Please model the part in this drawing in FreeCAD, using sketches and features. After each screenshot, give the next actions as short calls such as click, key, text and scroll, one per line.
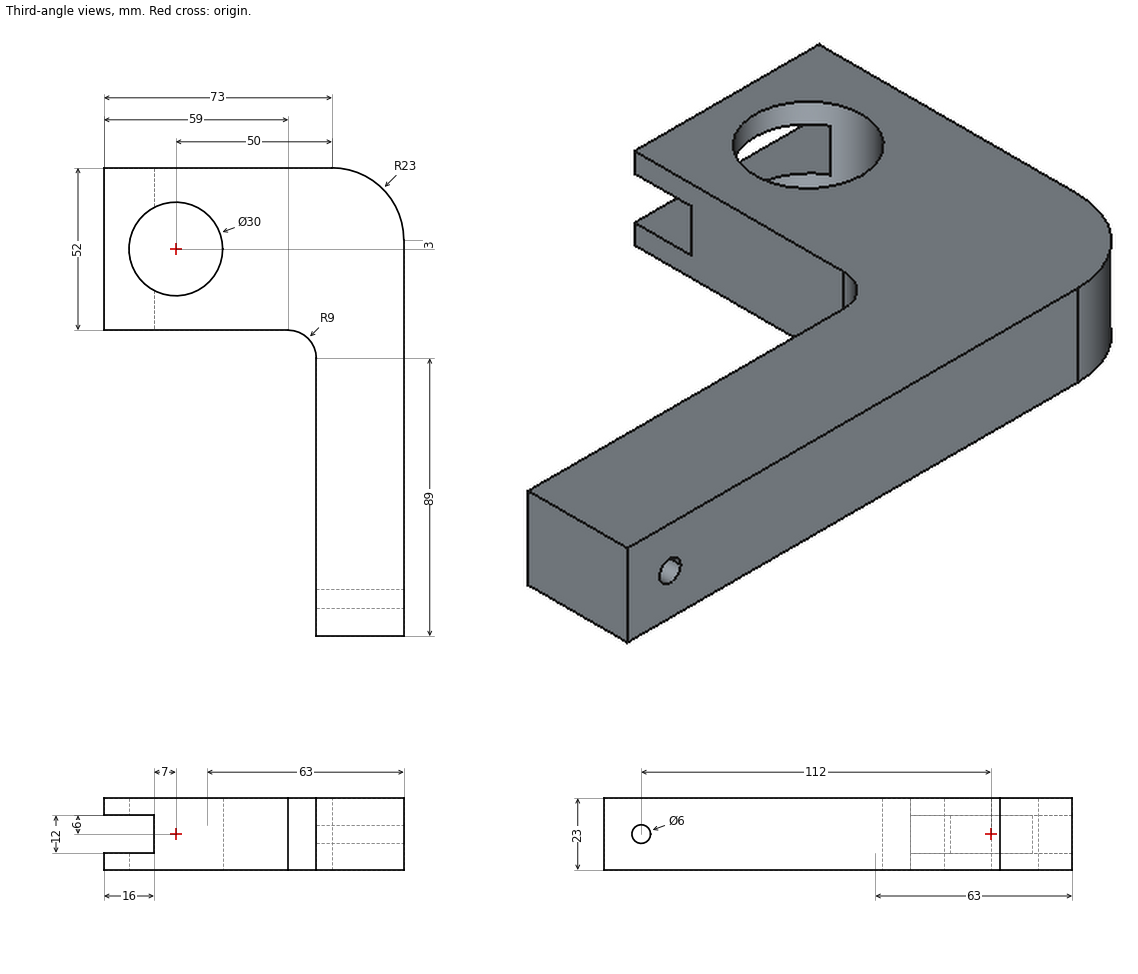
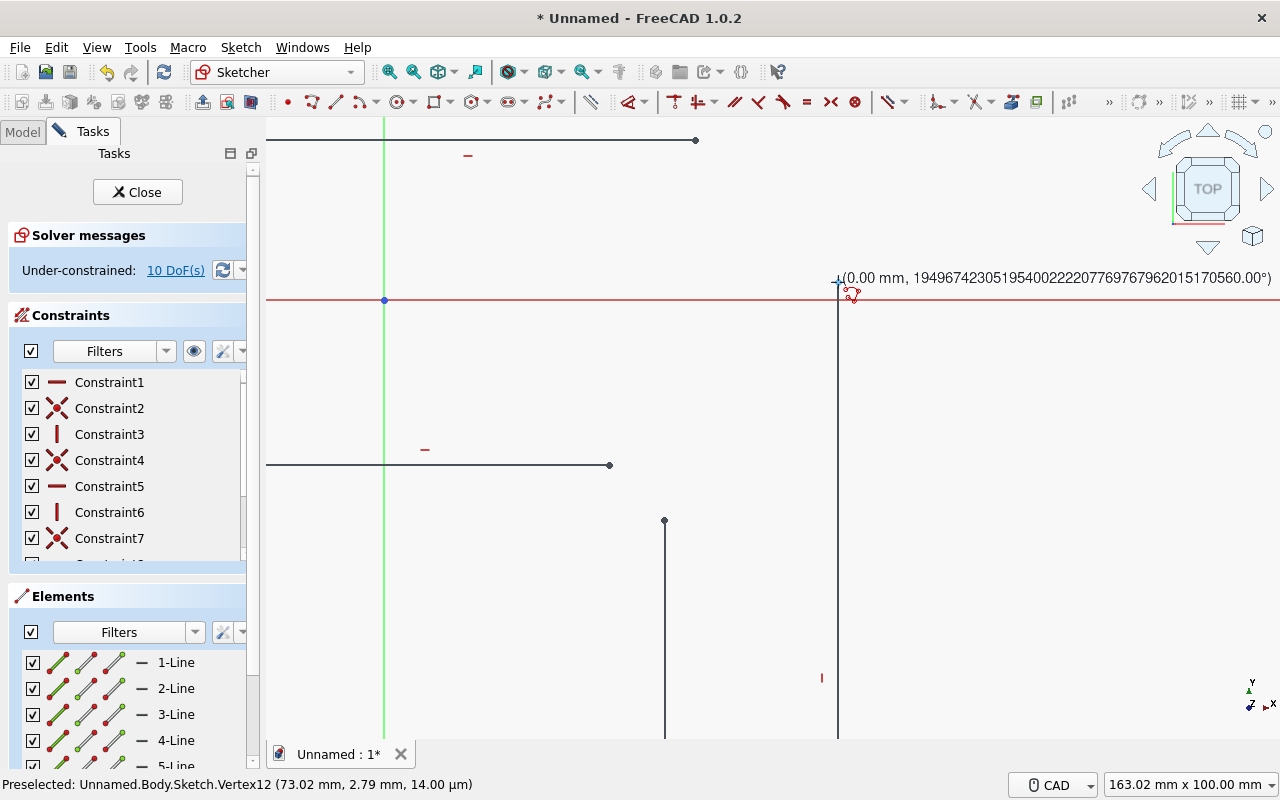
click(378, 102)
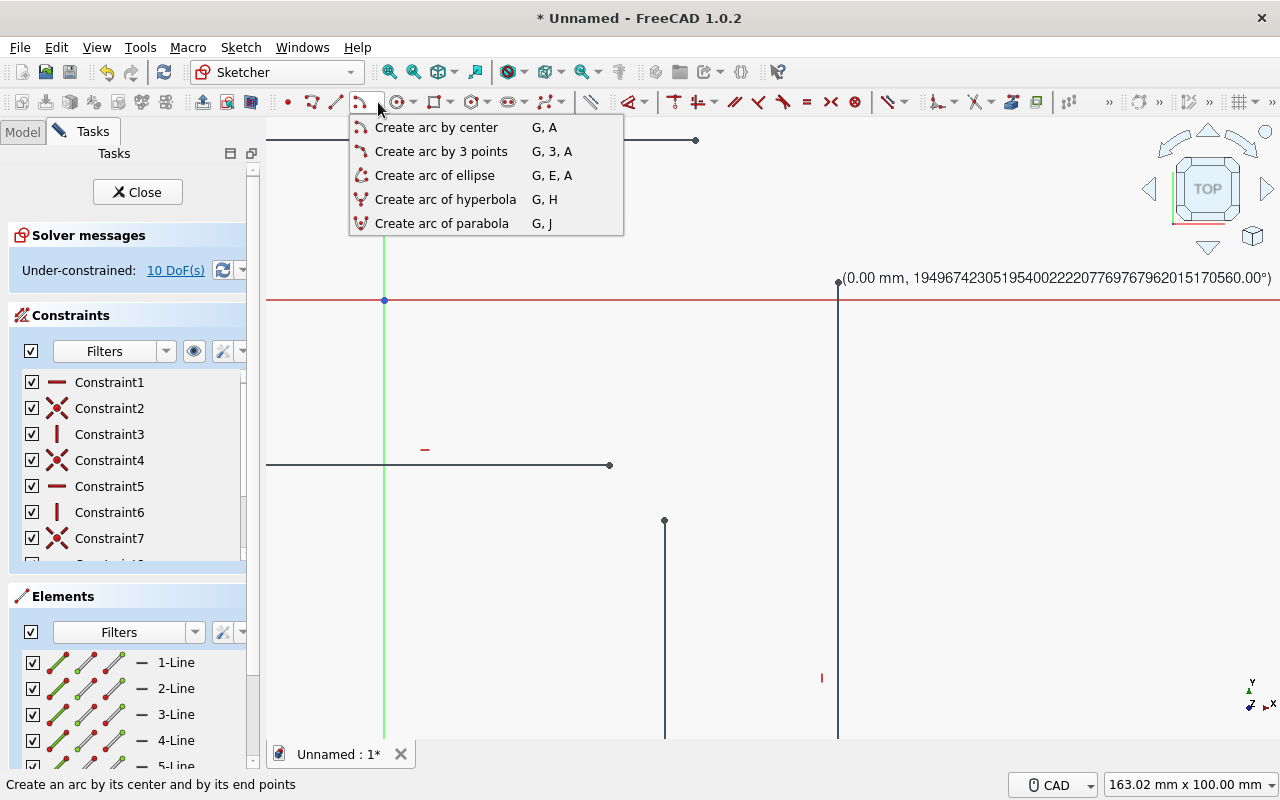
click(486, 151)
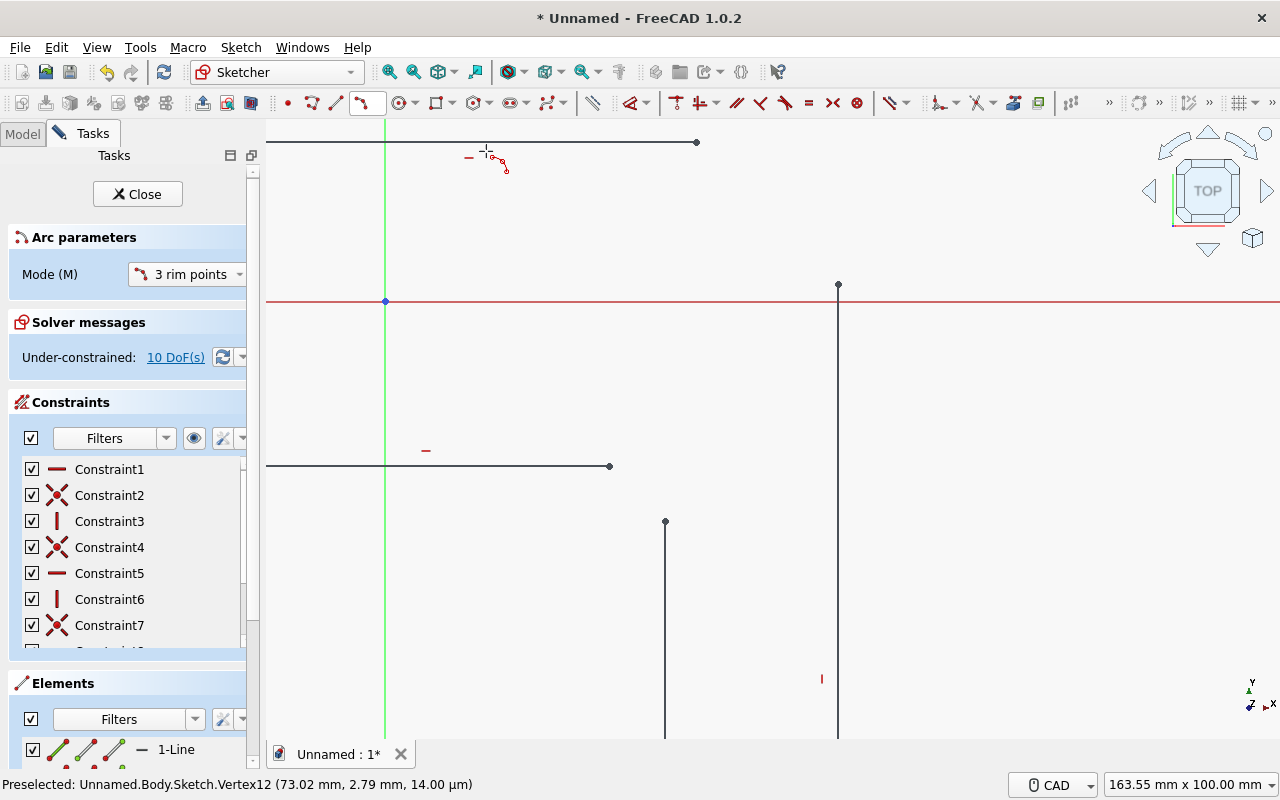
click(610, 466)
click(665, 522)
click(648, 479)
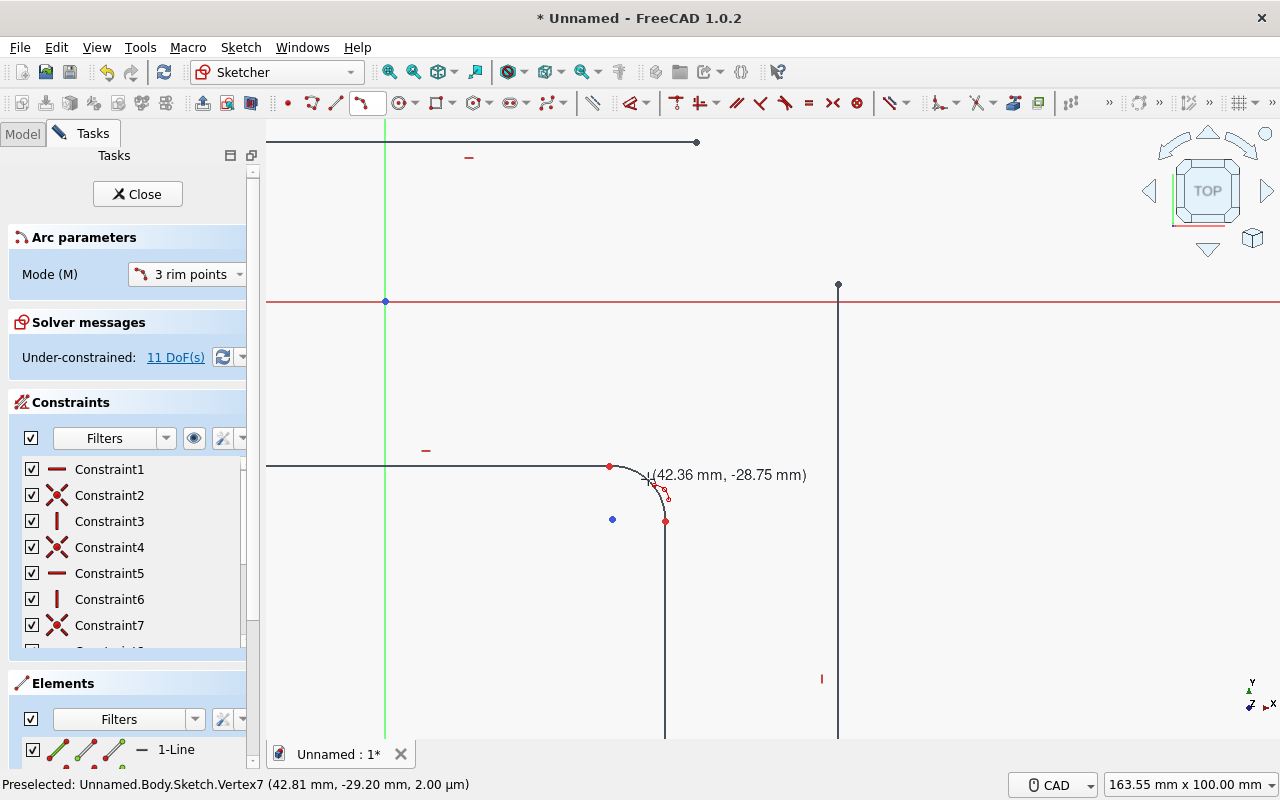
click(838, 284)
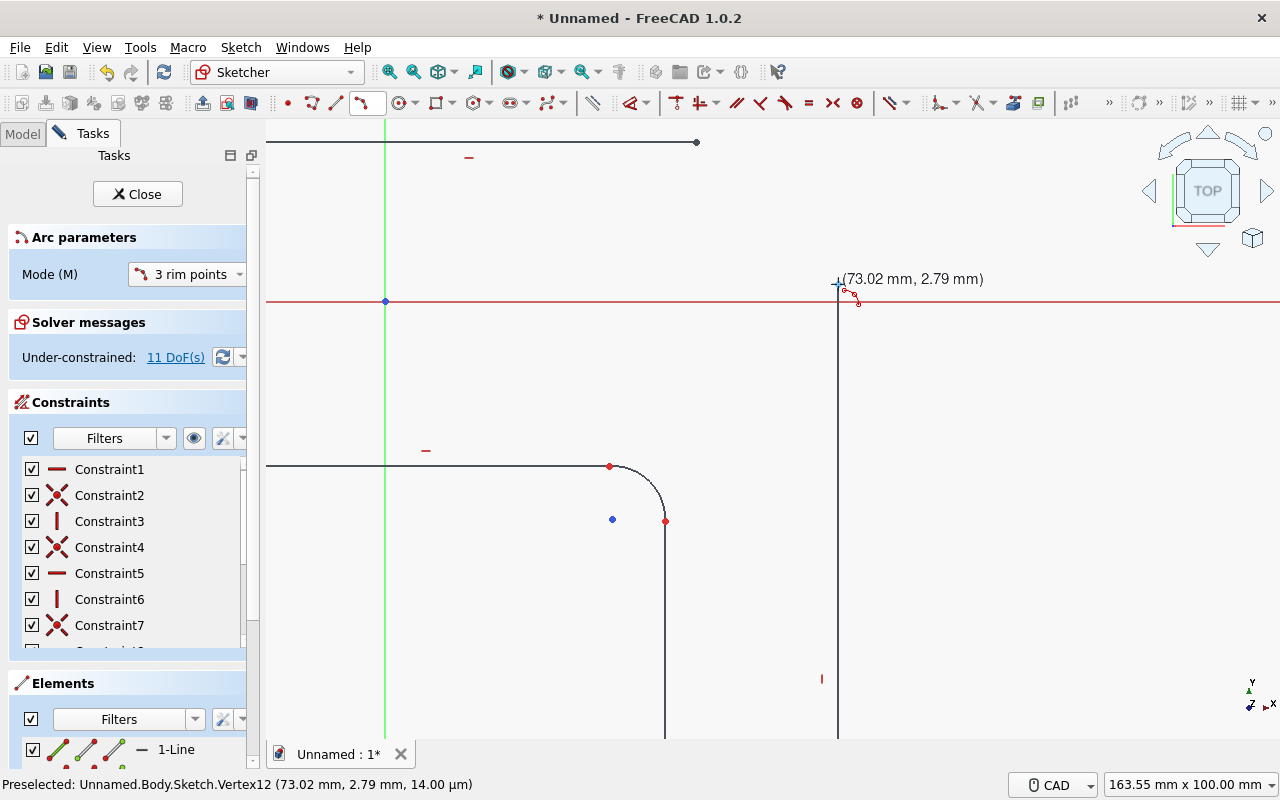
scroll(838, 285, down, 4)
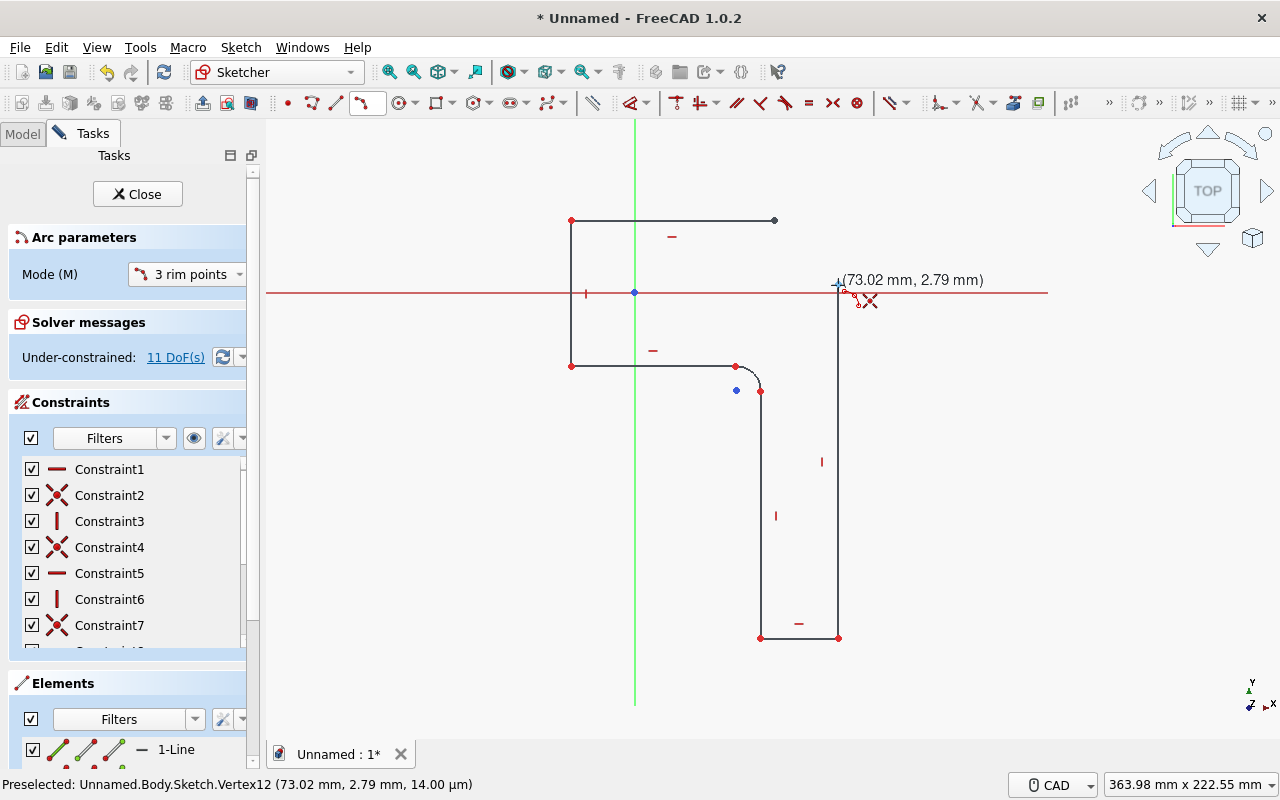
click(775, 221)
click(820, 239)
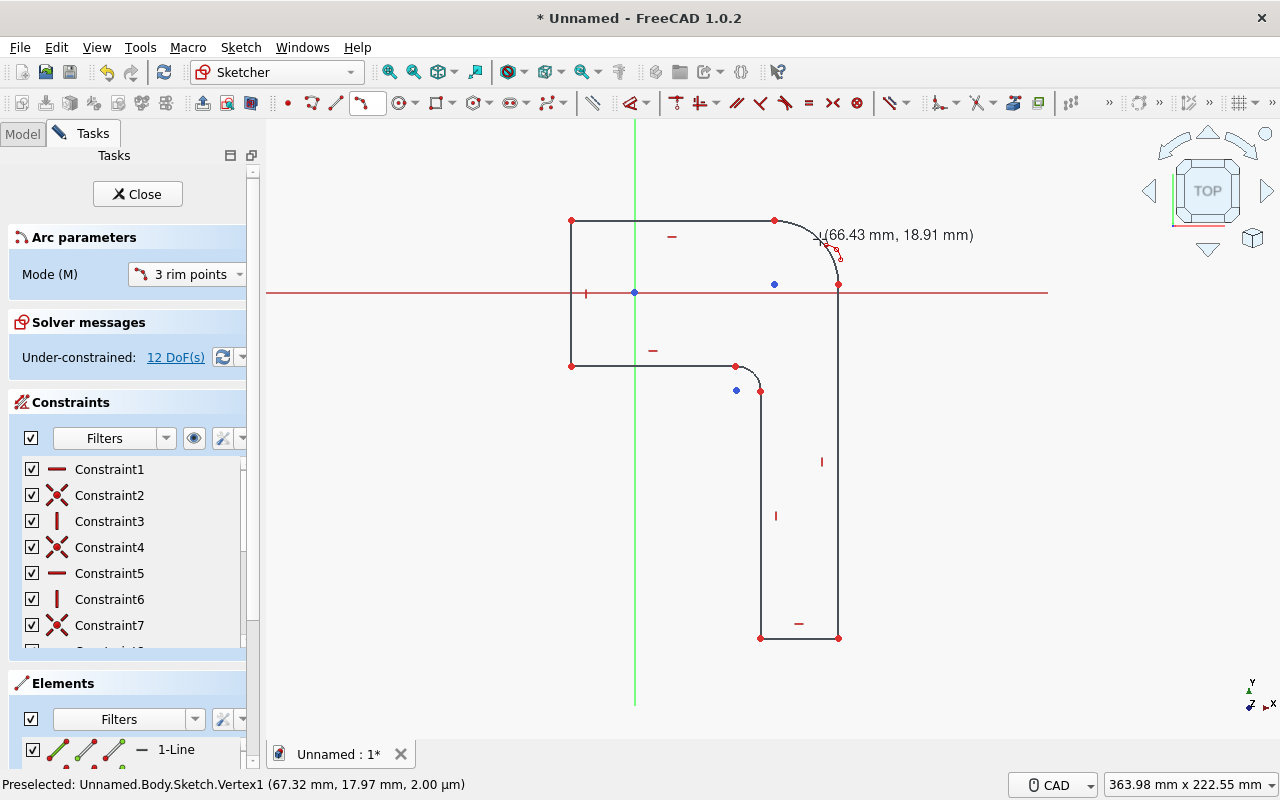
click(400, 104)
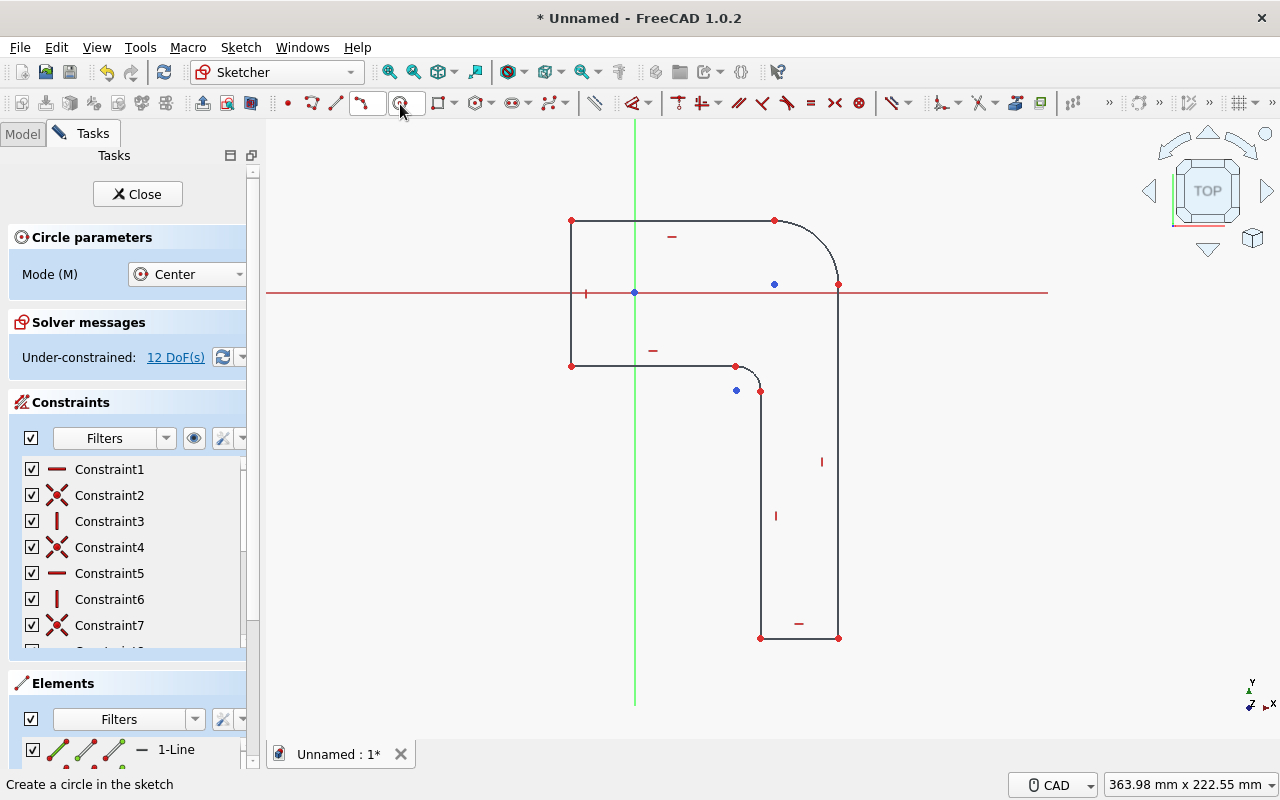
click(635, 293)
move(664, 263)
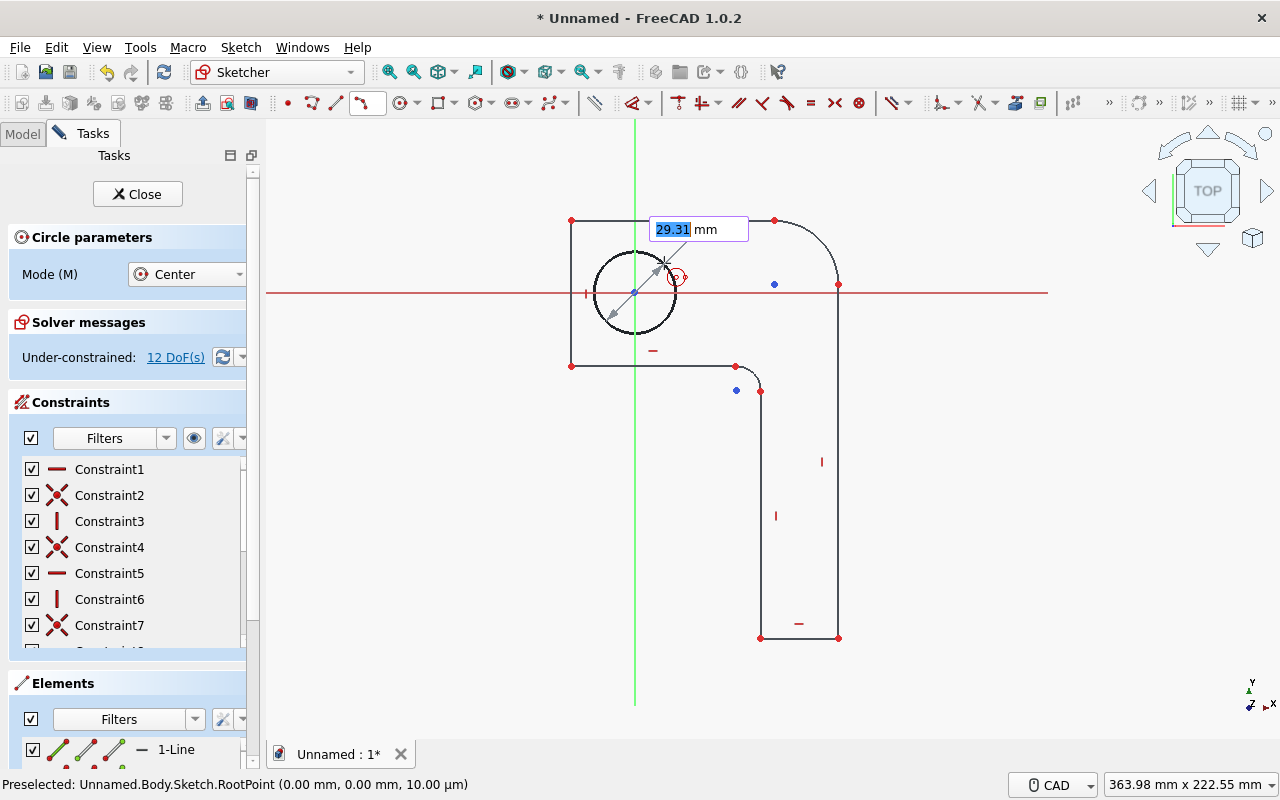
text(30)
key(Return)
key(Escape)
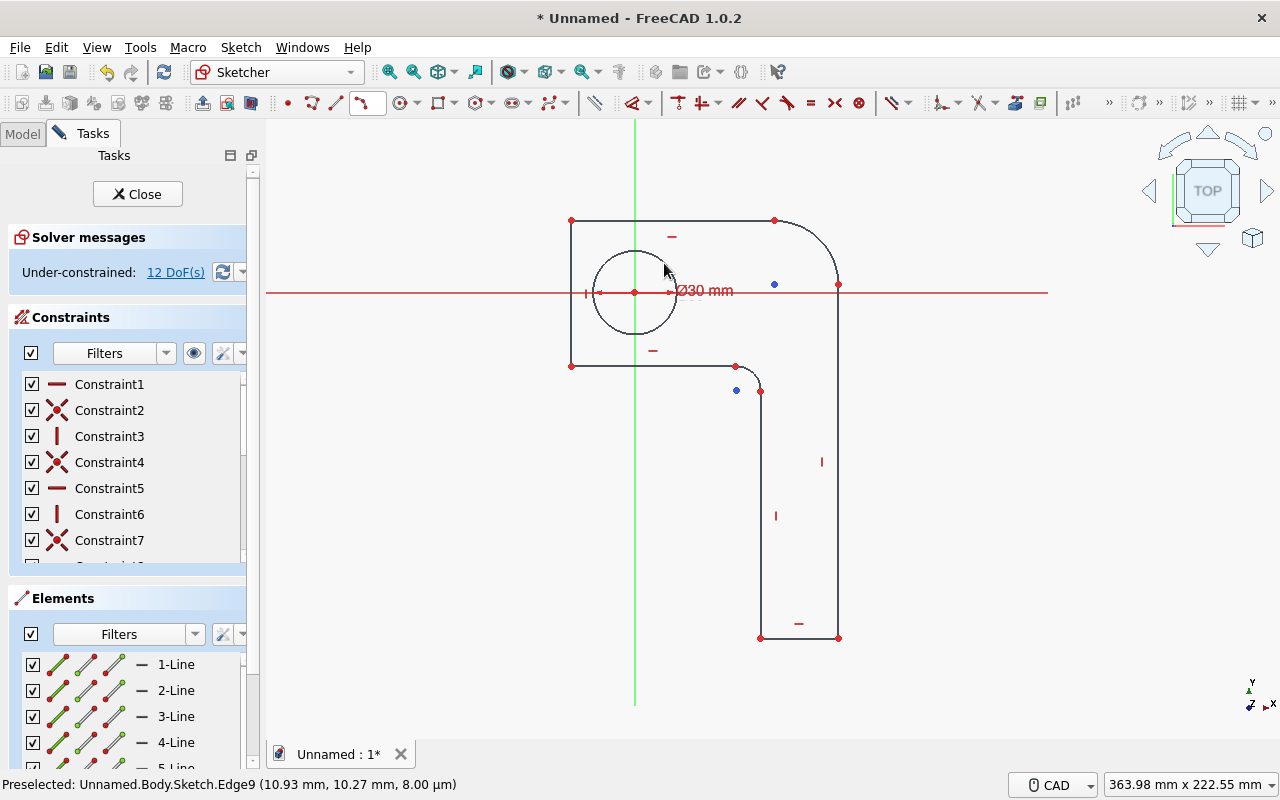
click(714, 221)